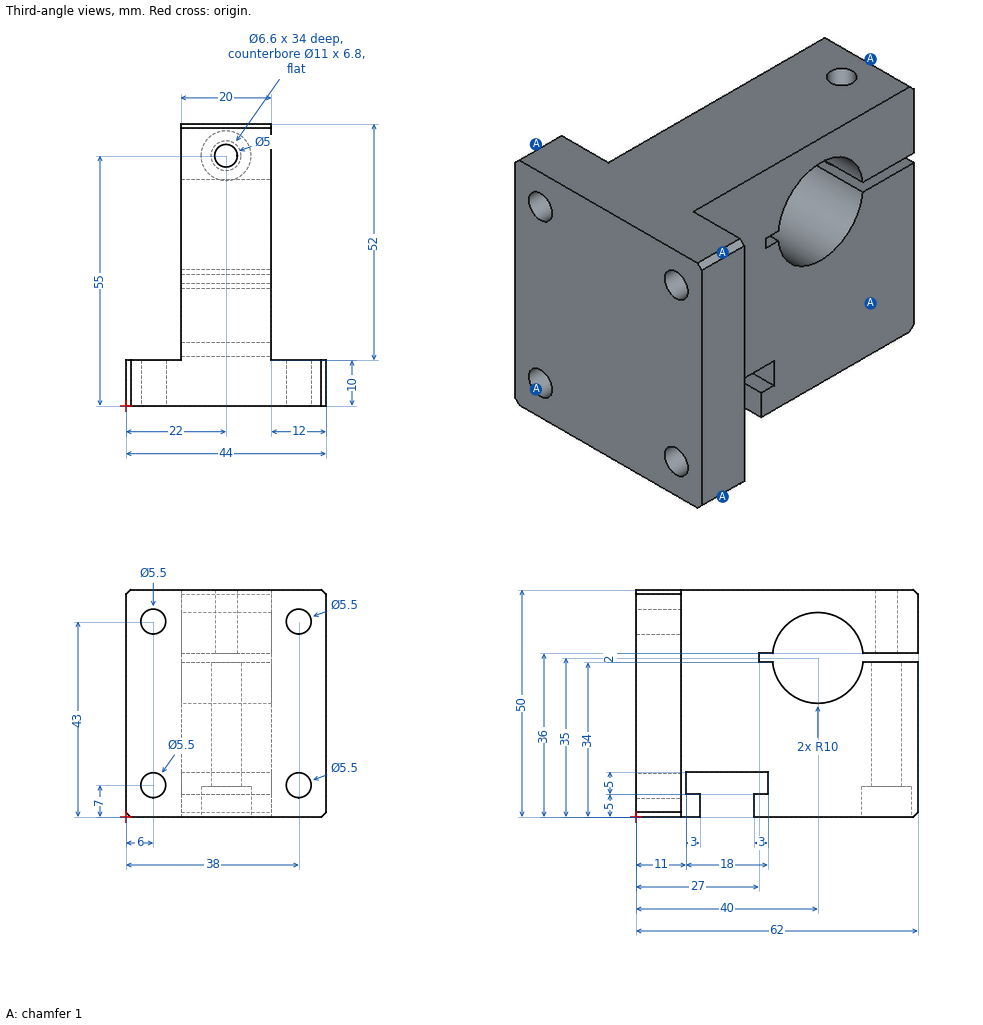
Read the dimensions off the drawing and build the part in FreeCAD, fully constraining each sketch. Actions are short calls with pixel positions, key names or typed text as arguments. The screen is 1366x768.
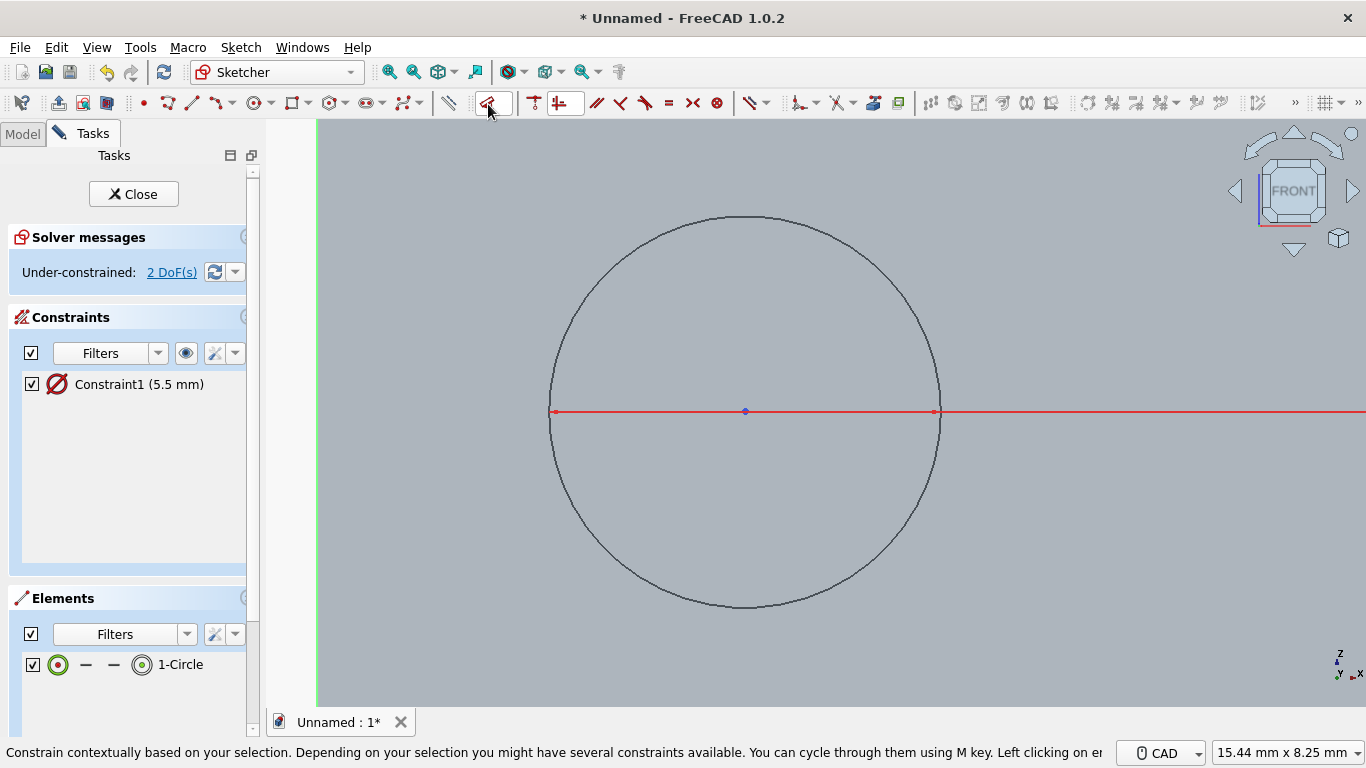
click(745, 412)
click(531, 378)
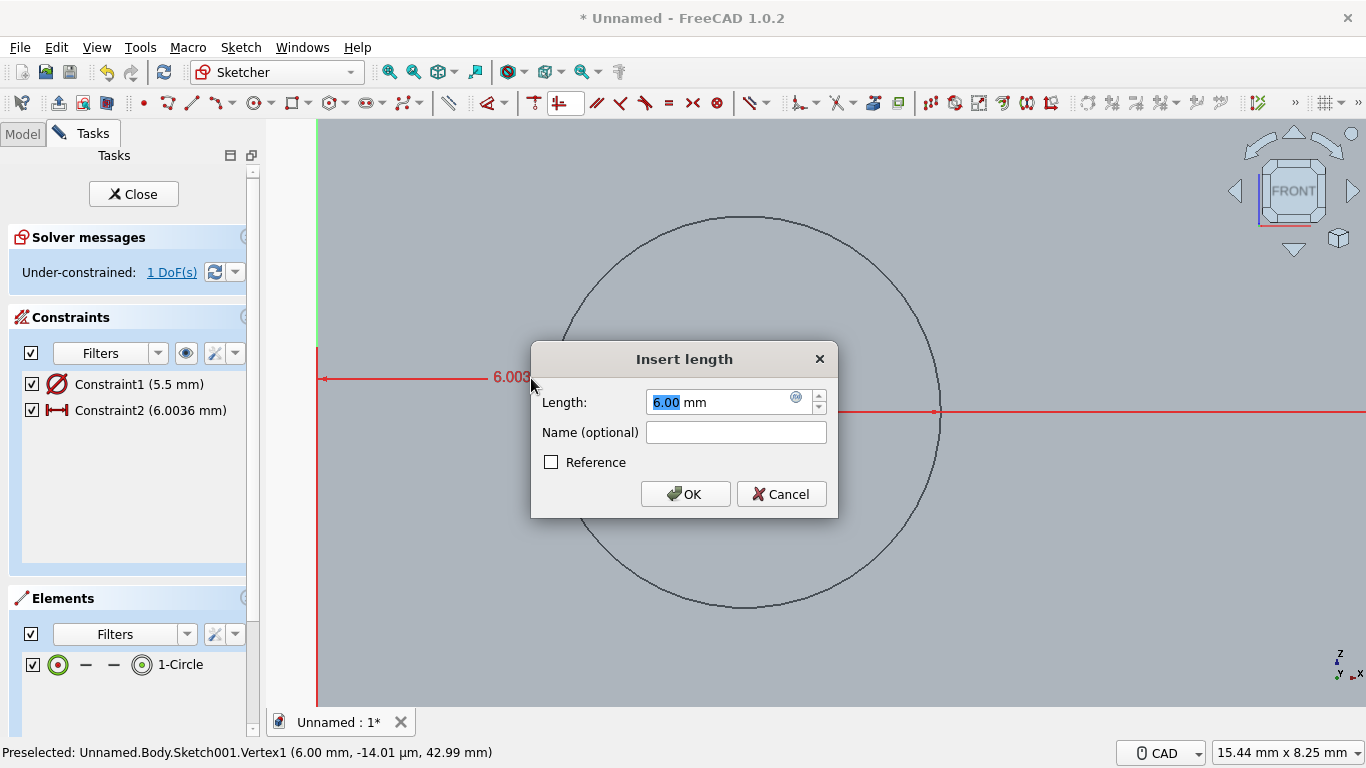
text(6)
key(Return)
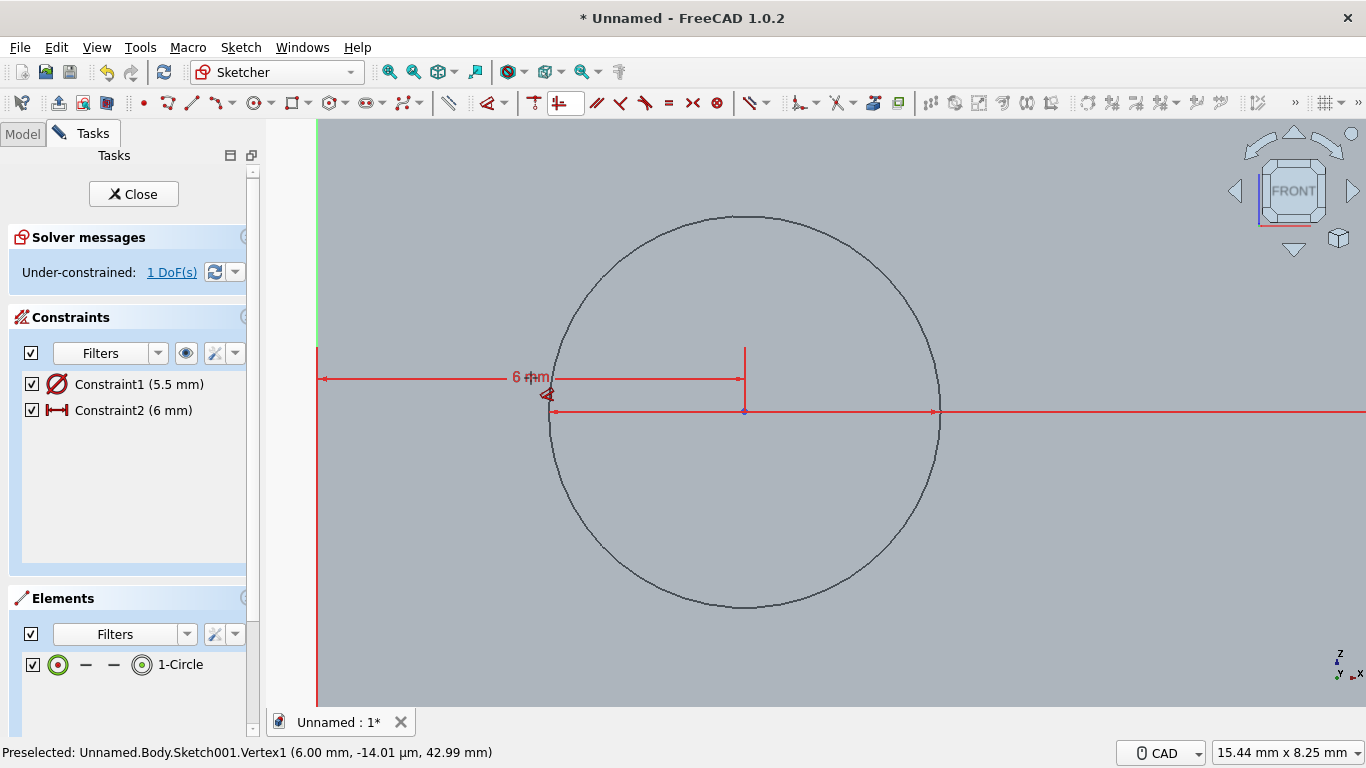
click(745, 412)
click(779, 546)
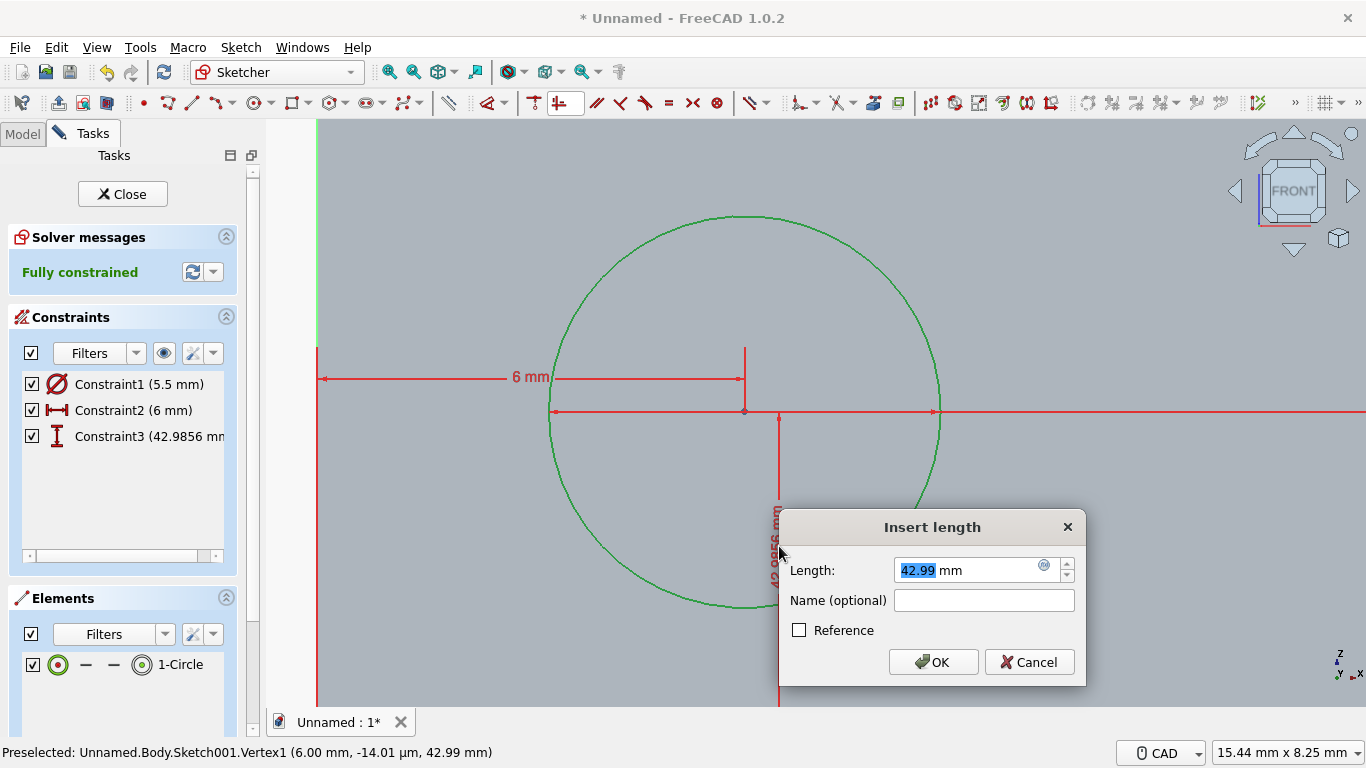
text(43)
key(Return)
key(Escape)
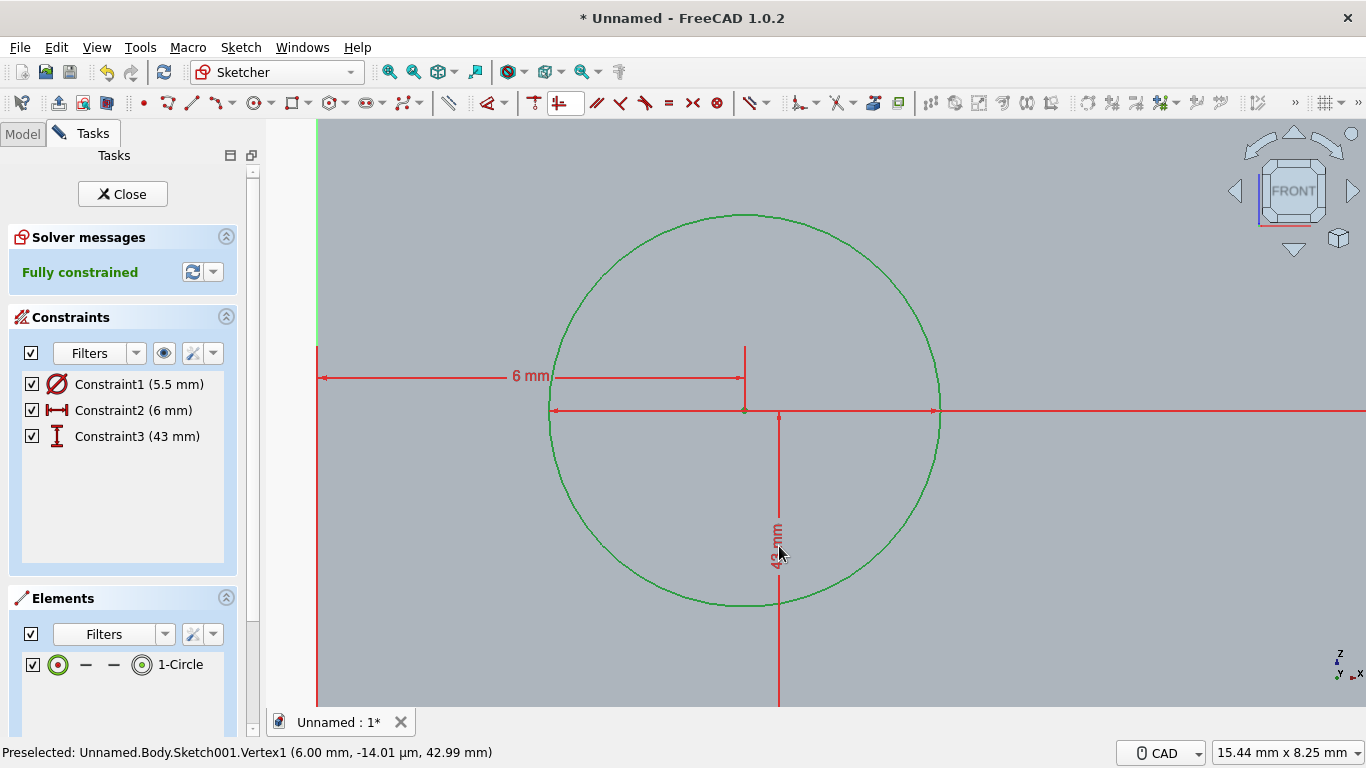
click(123, 194)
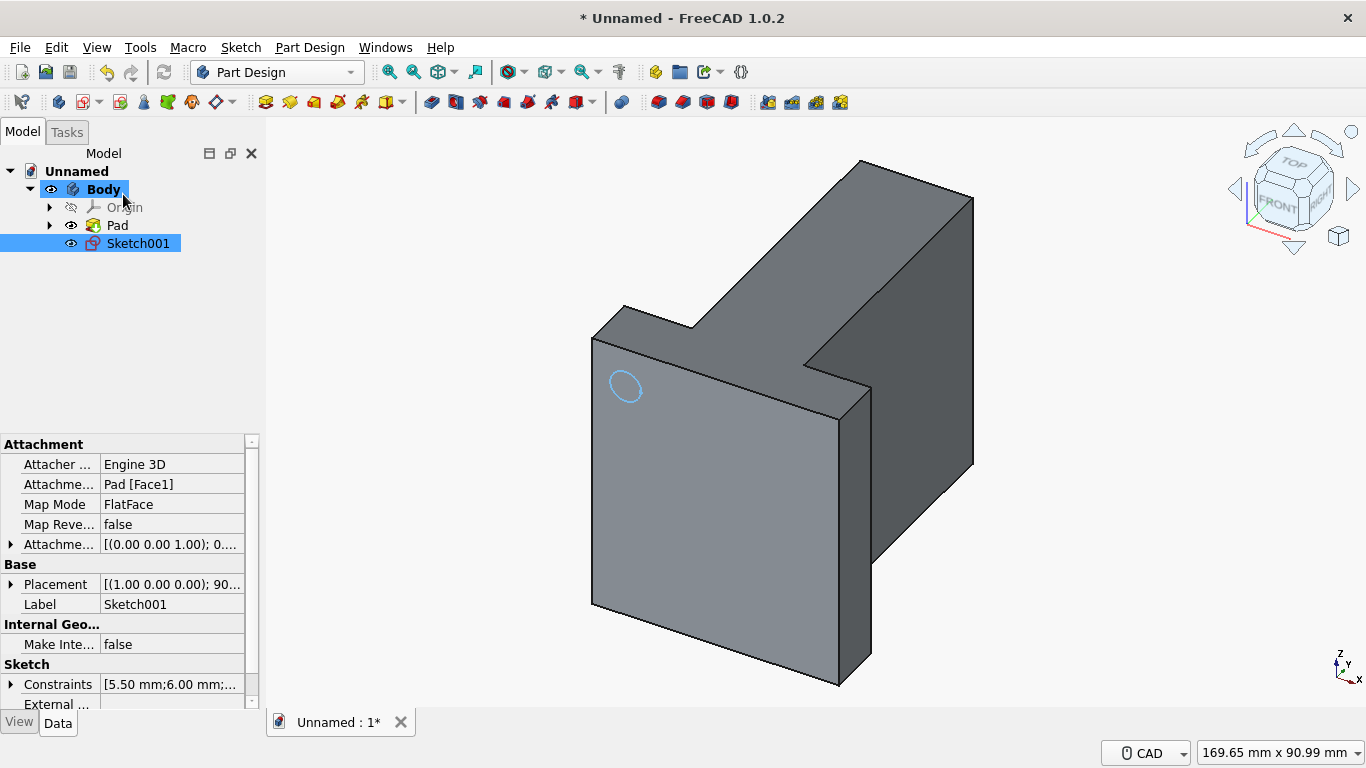
click(432, 102)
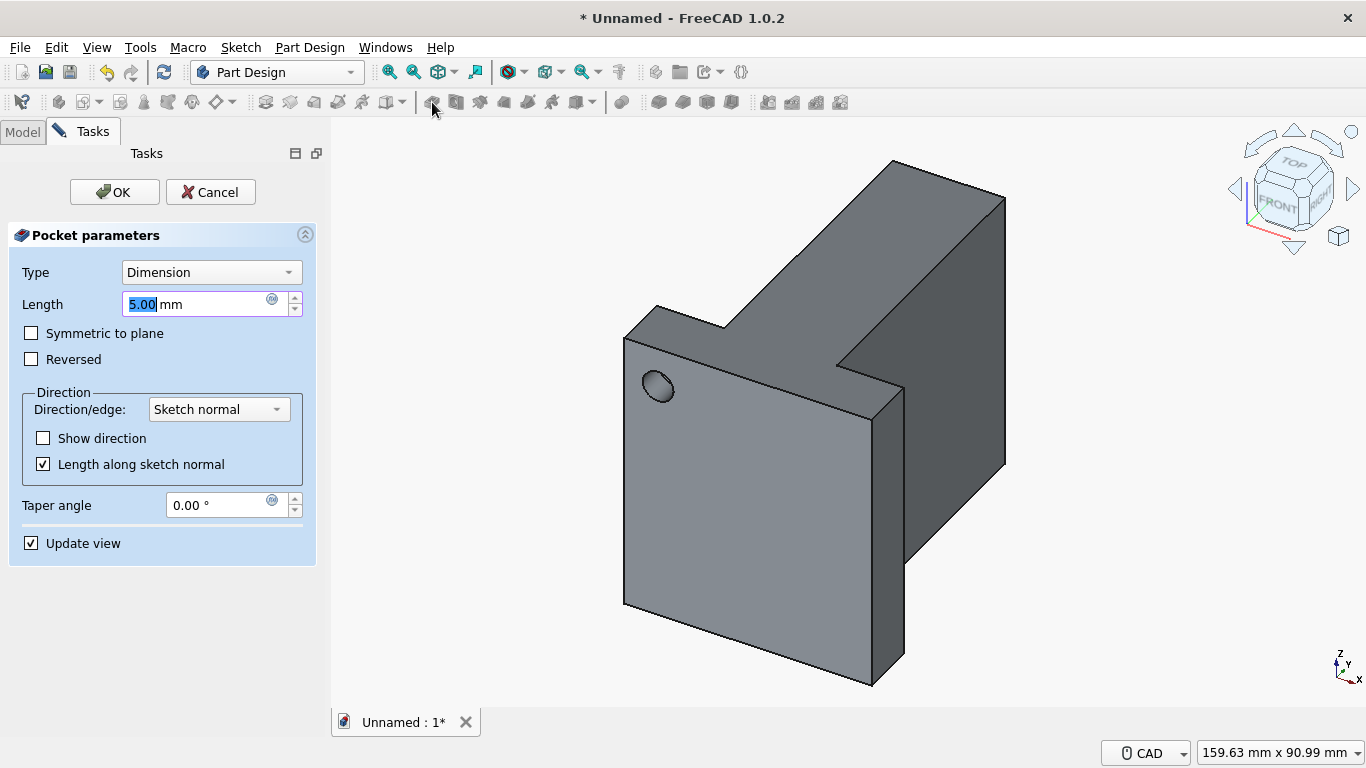
click(212, 272)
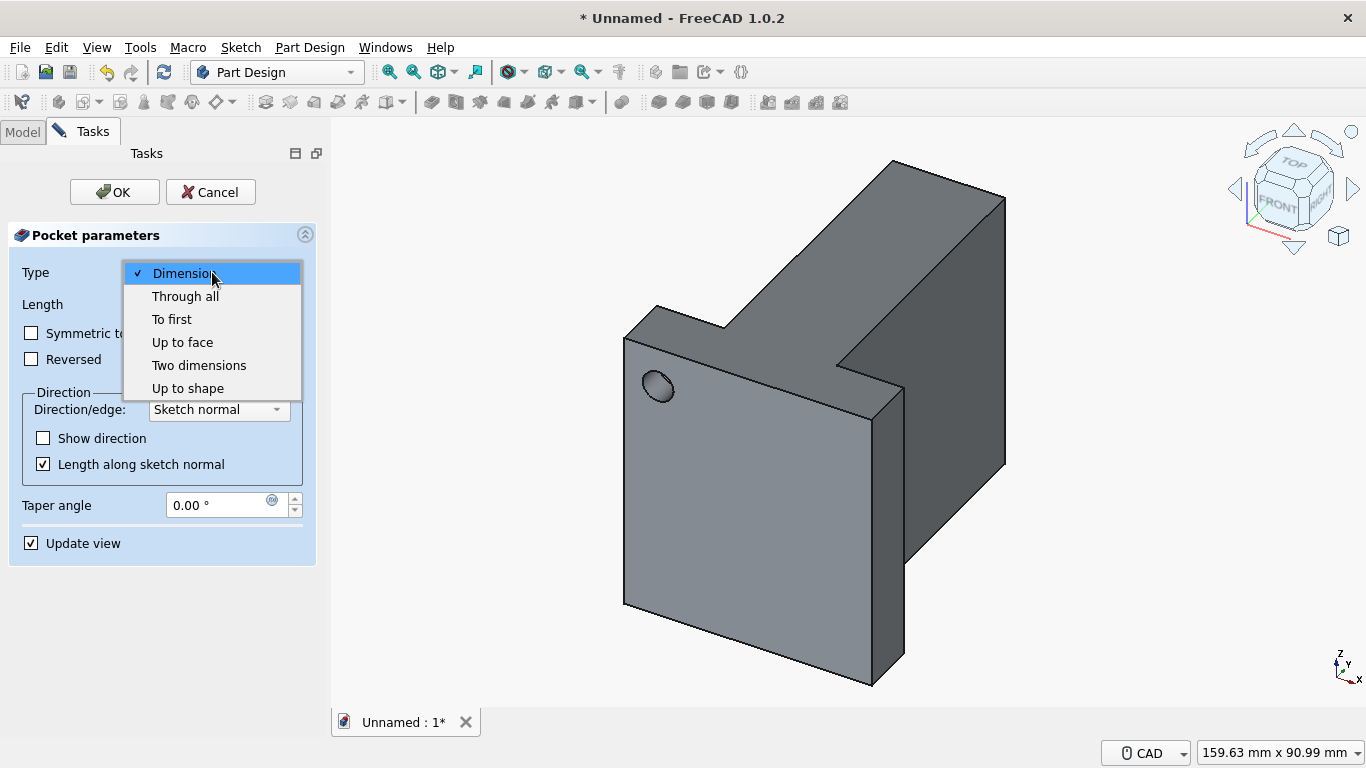
click(212, 320)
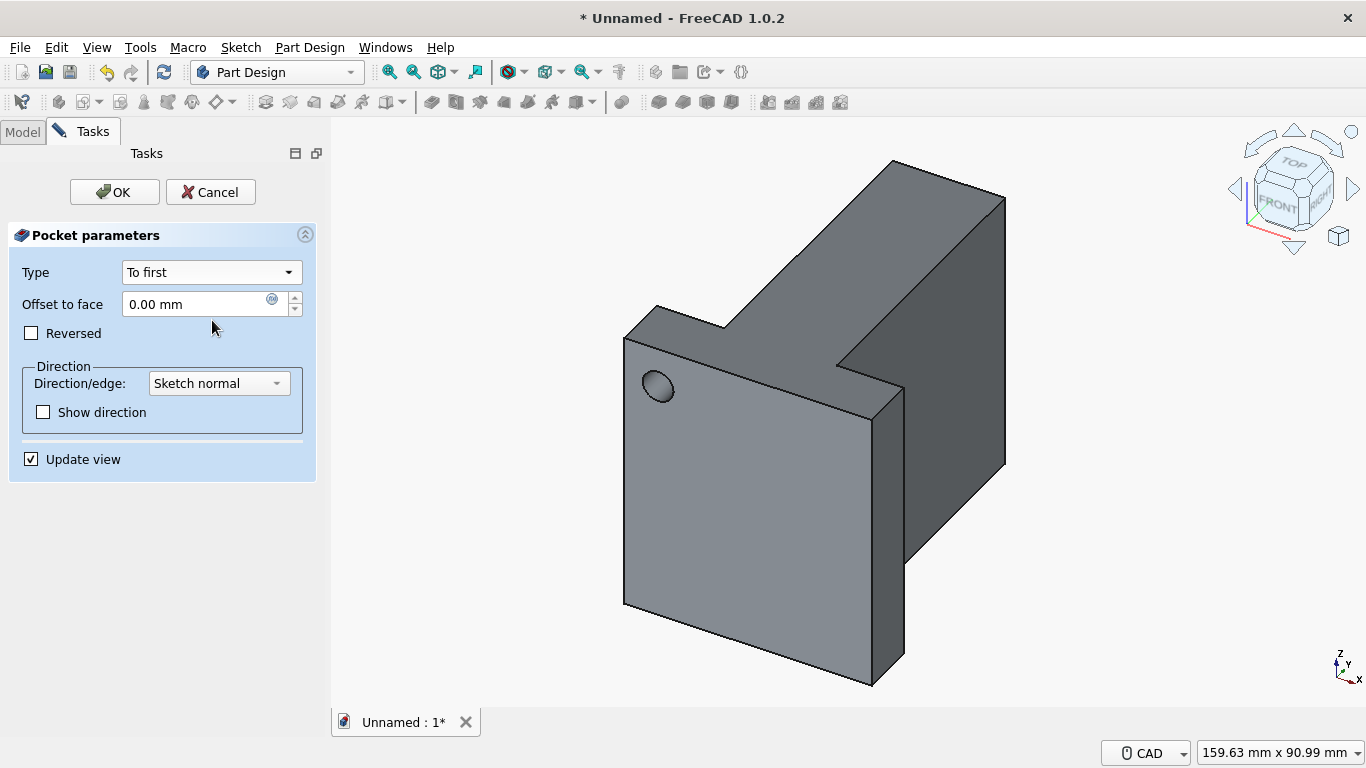
click(115, 192)